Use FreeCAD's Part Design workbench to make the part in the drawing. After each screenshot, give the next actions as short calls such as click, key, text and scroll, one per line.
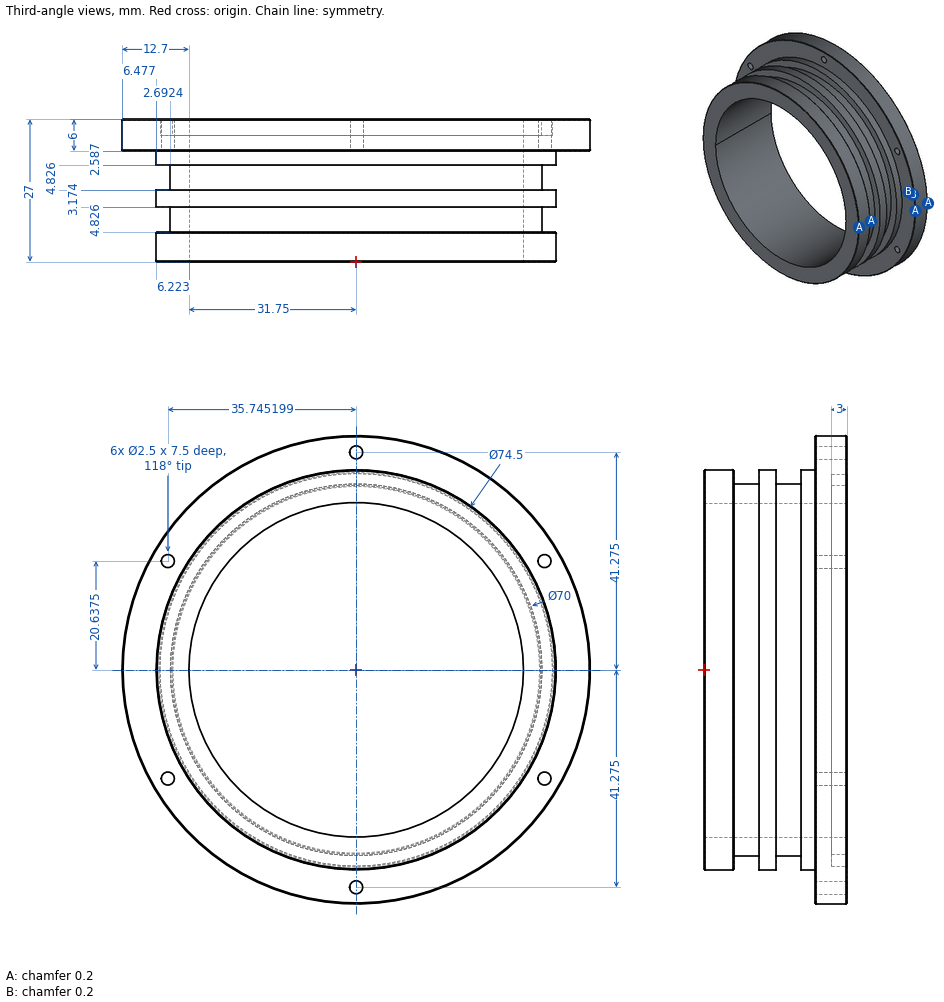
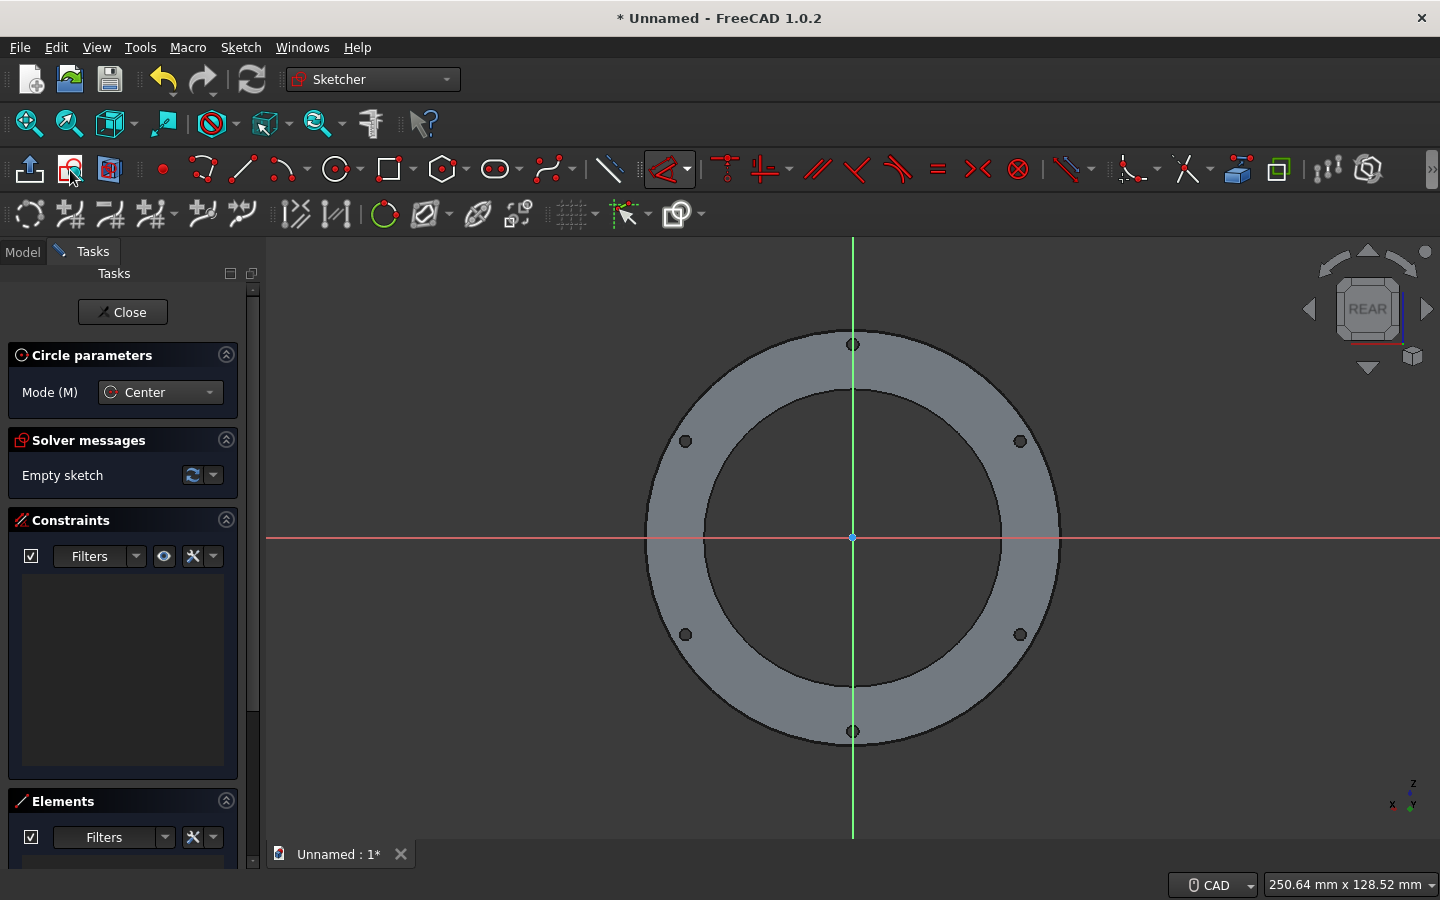
click(853, 538)
move(976, 415)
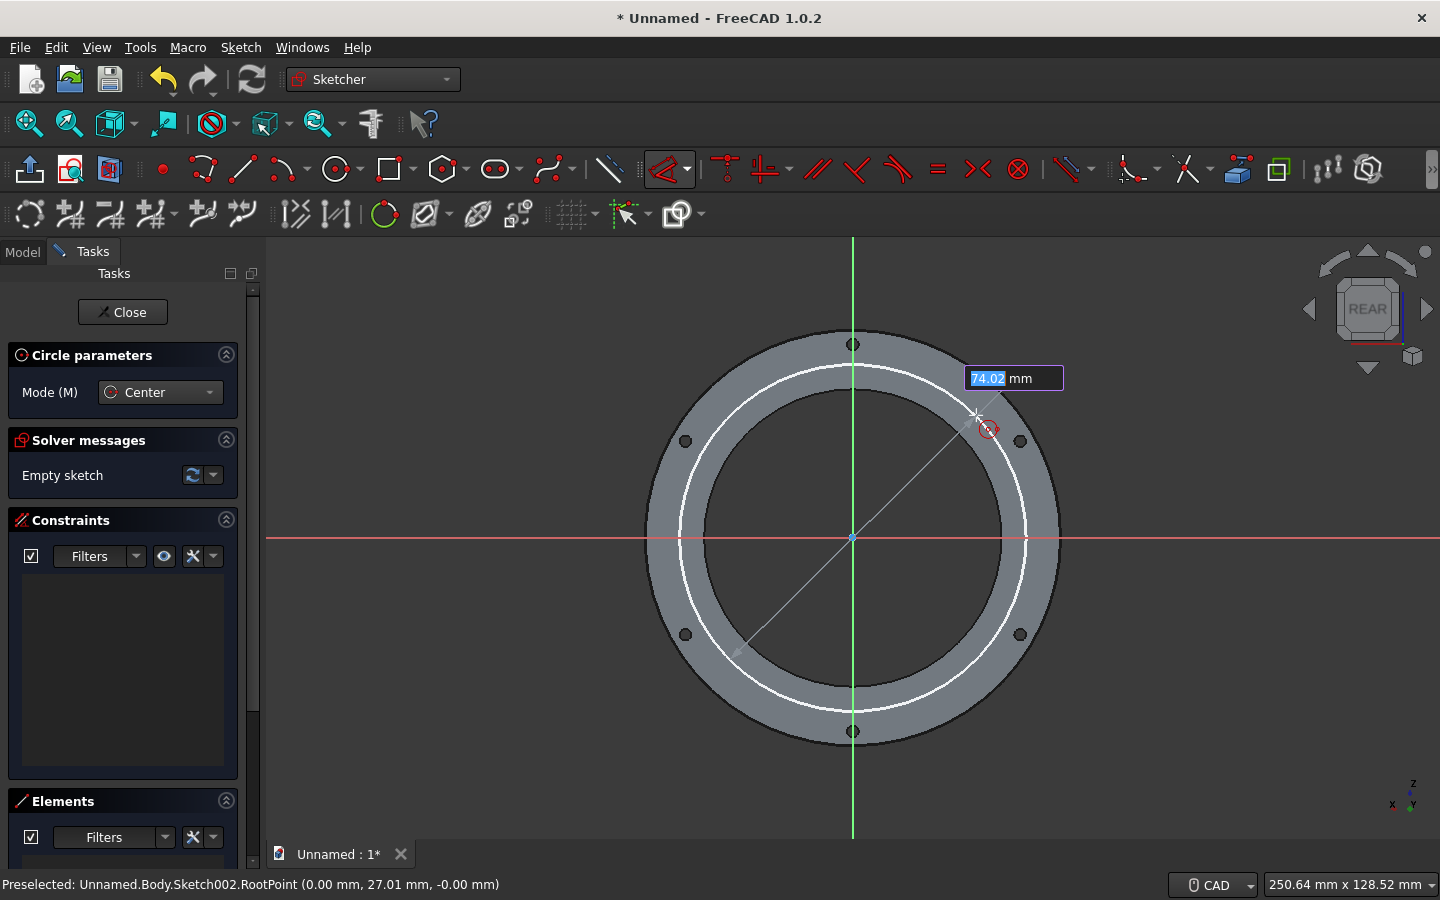
text(74.5)
key(Return)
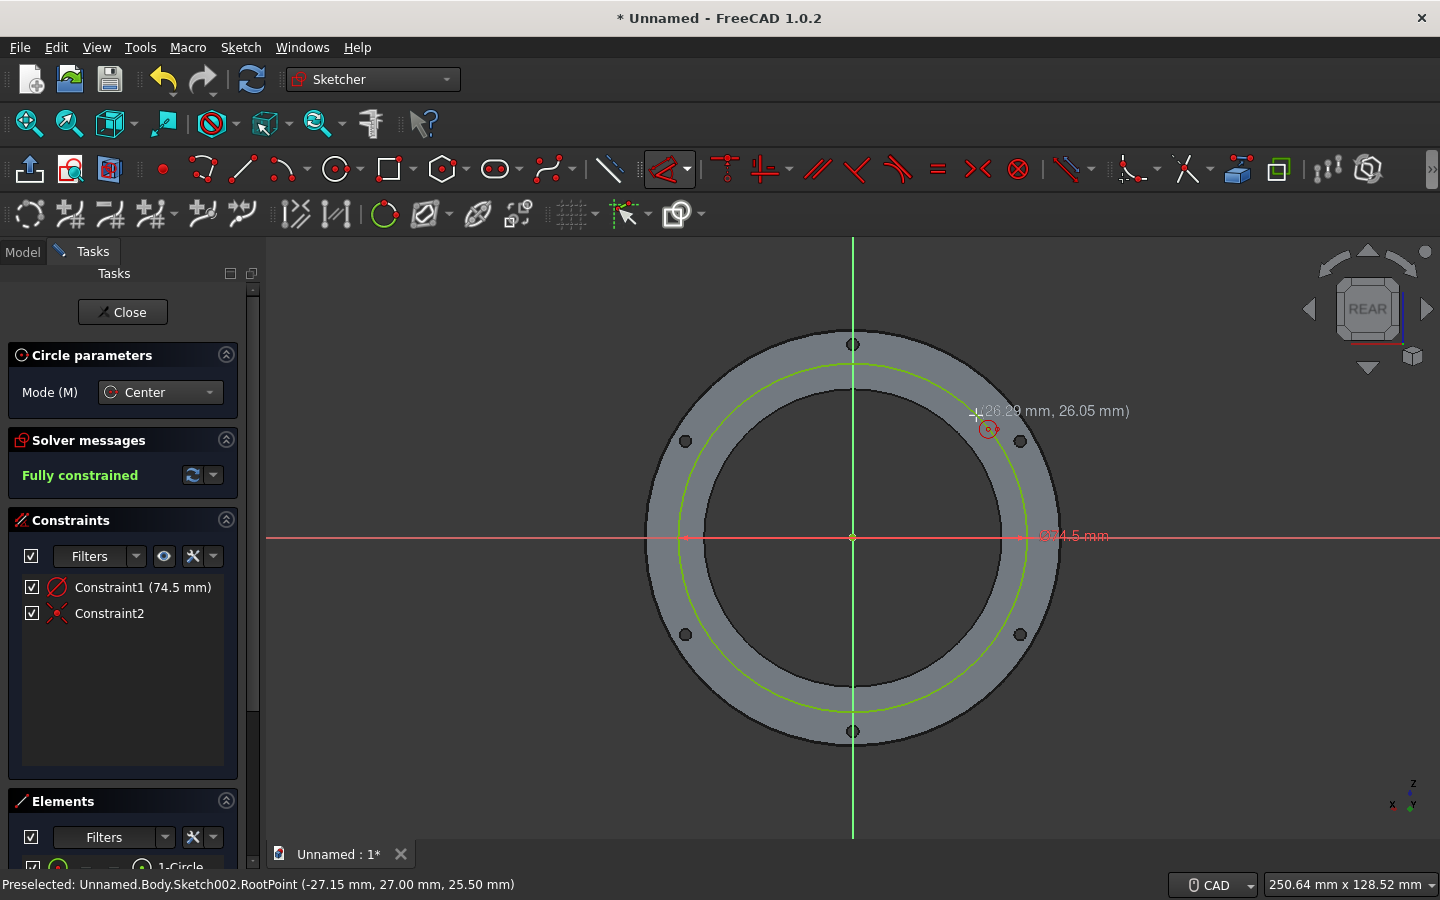
click(853, 538)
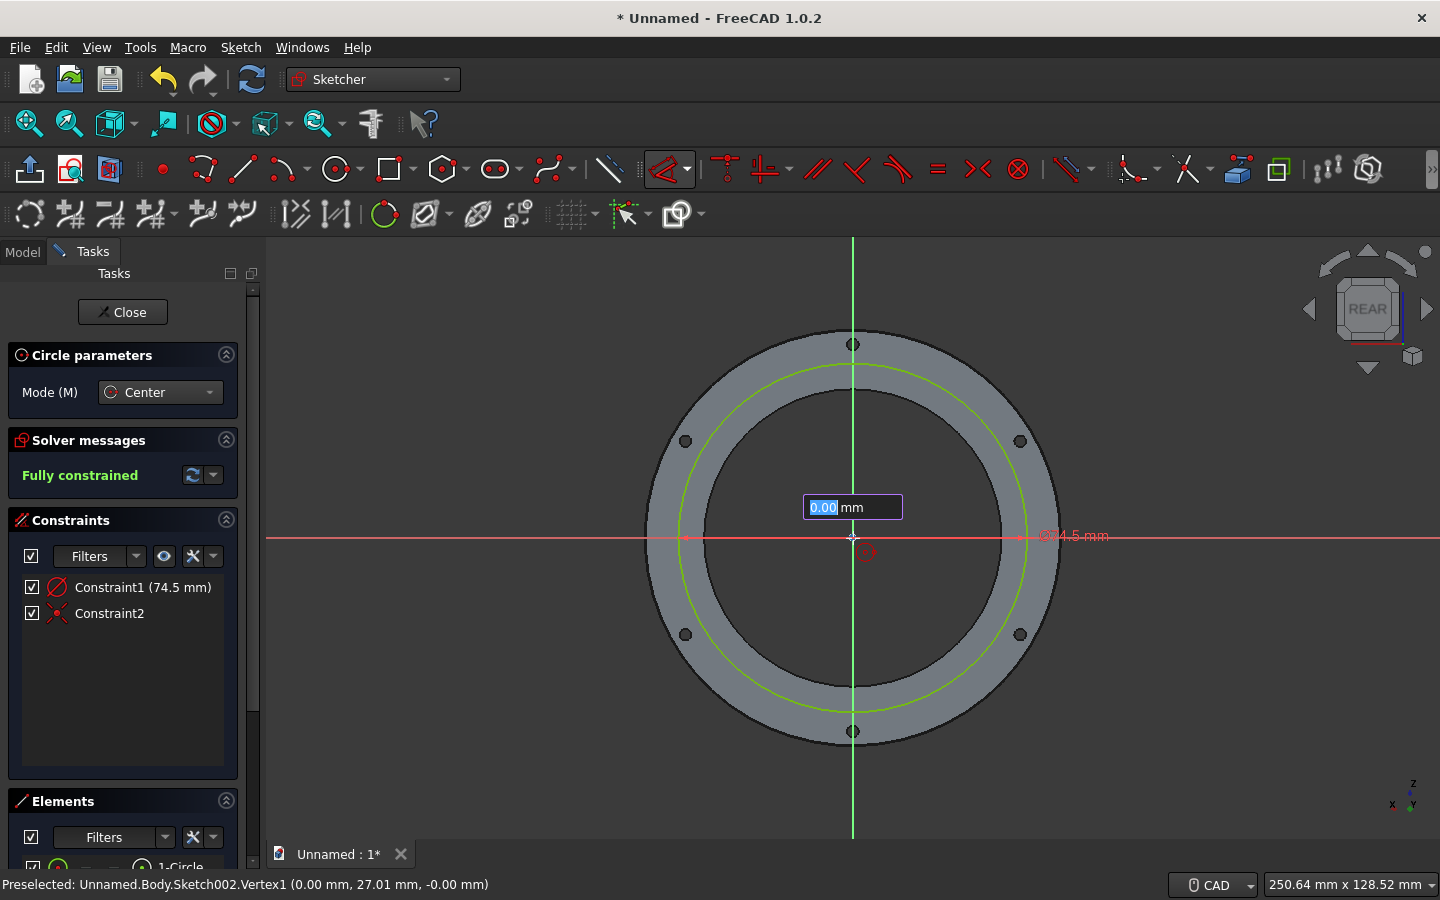
scroll(969, 422, up, 3)
move(968, 422)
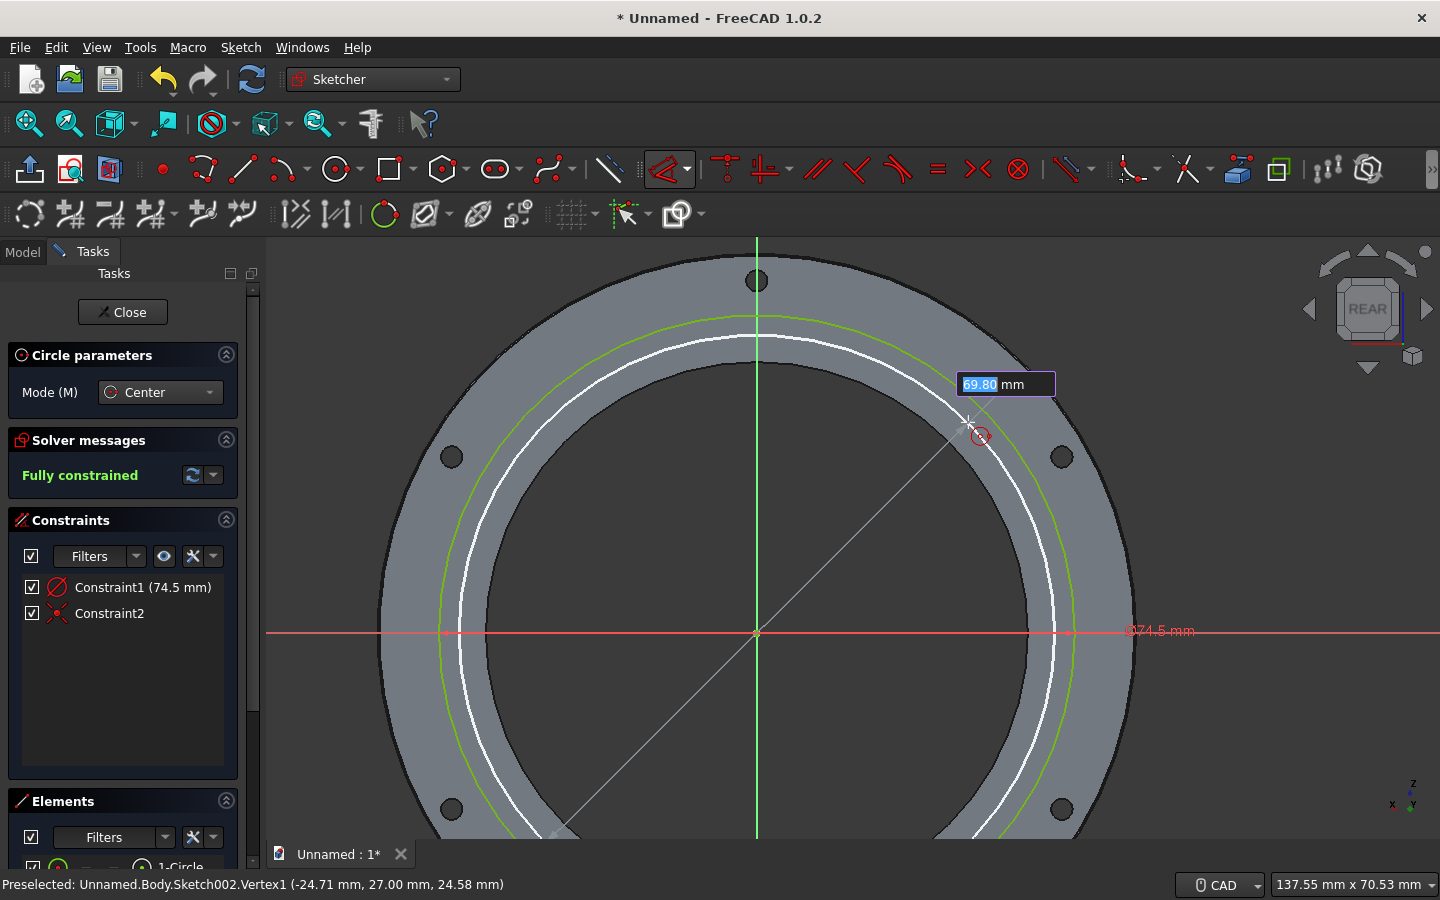
text(70)
key(Return)
key(Escape)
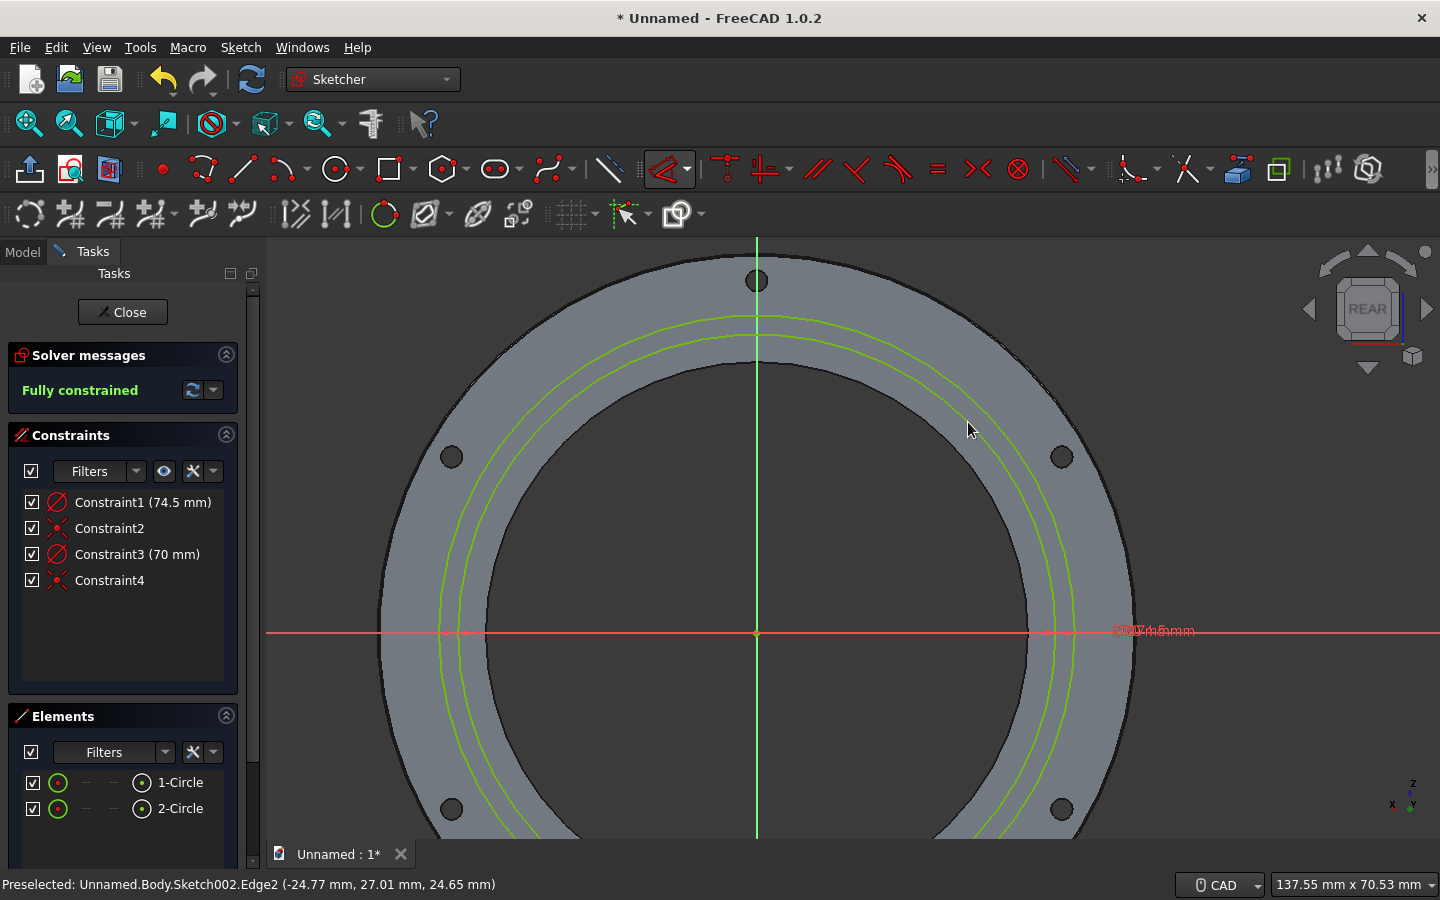
click(123, 312)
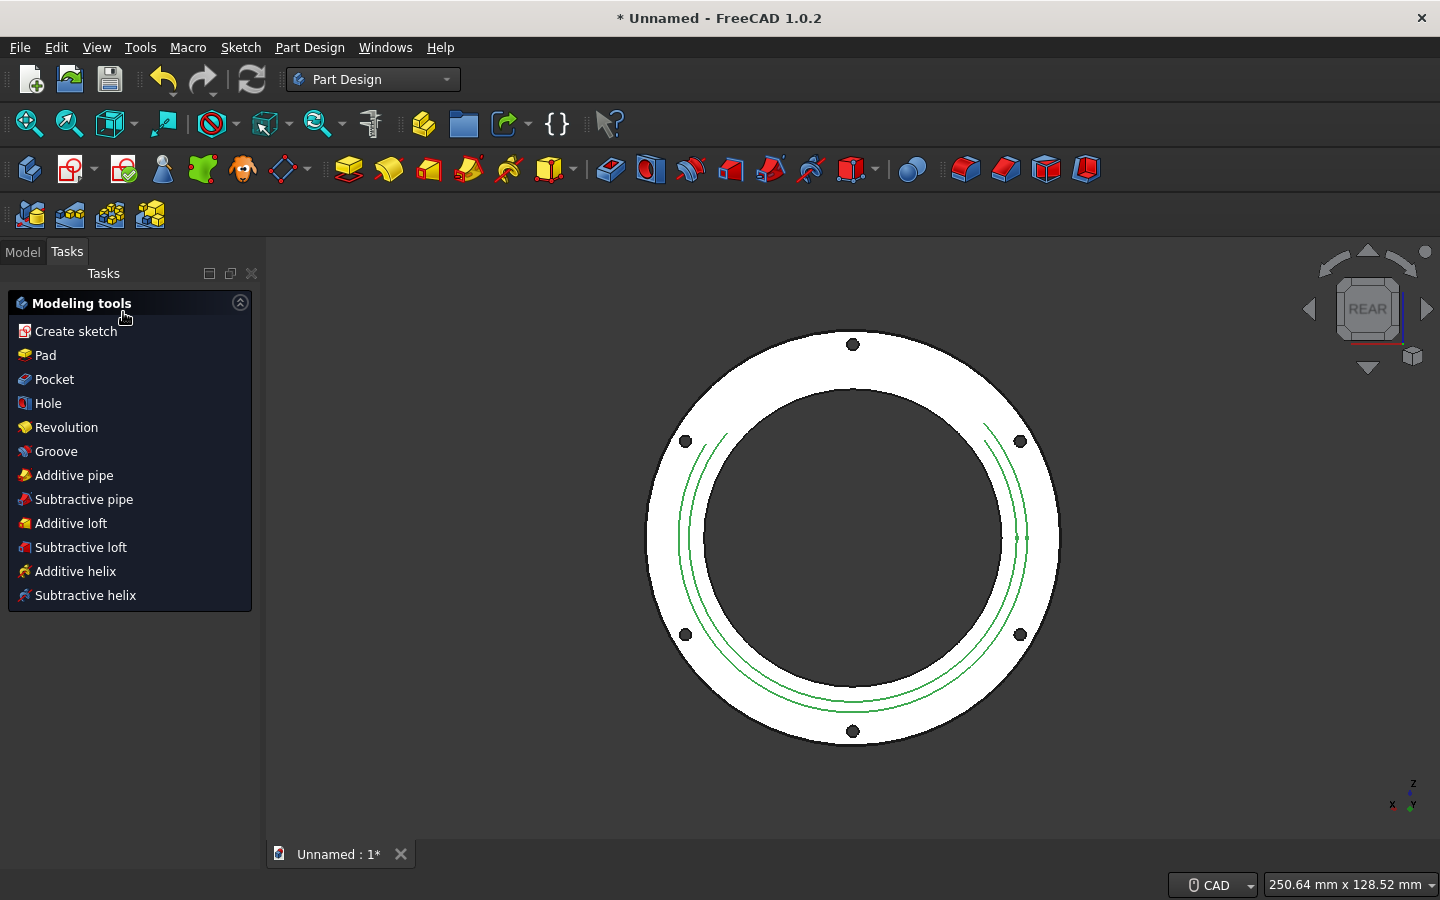
click(612, 170)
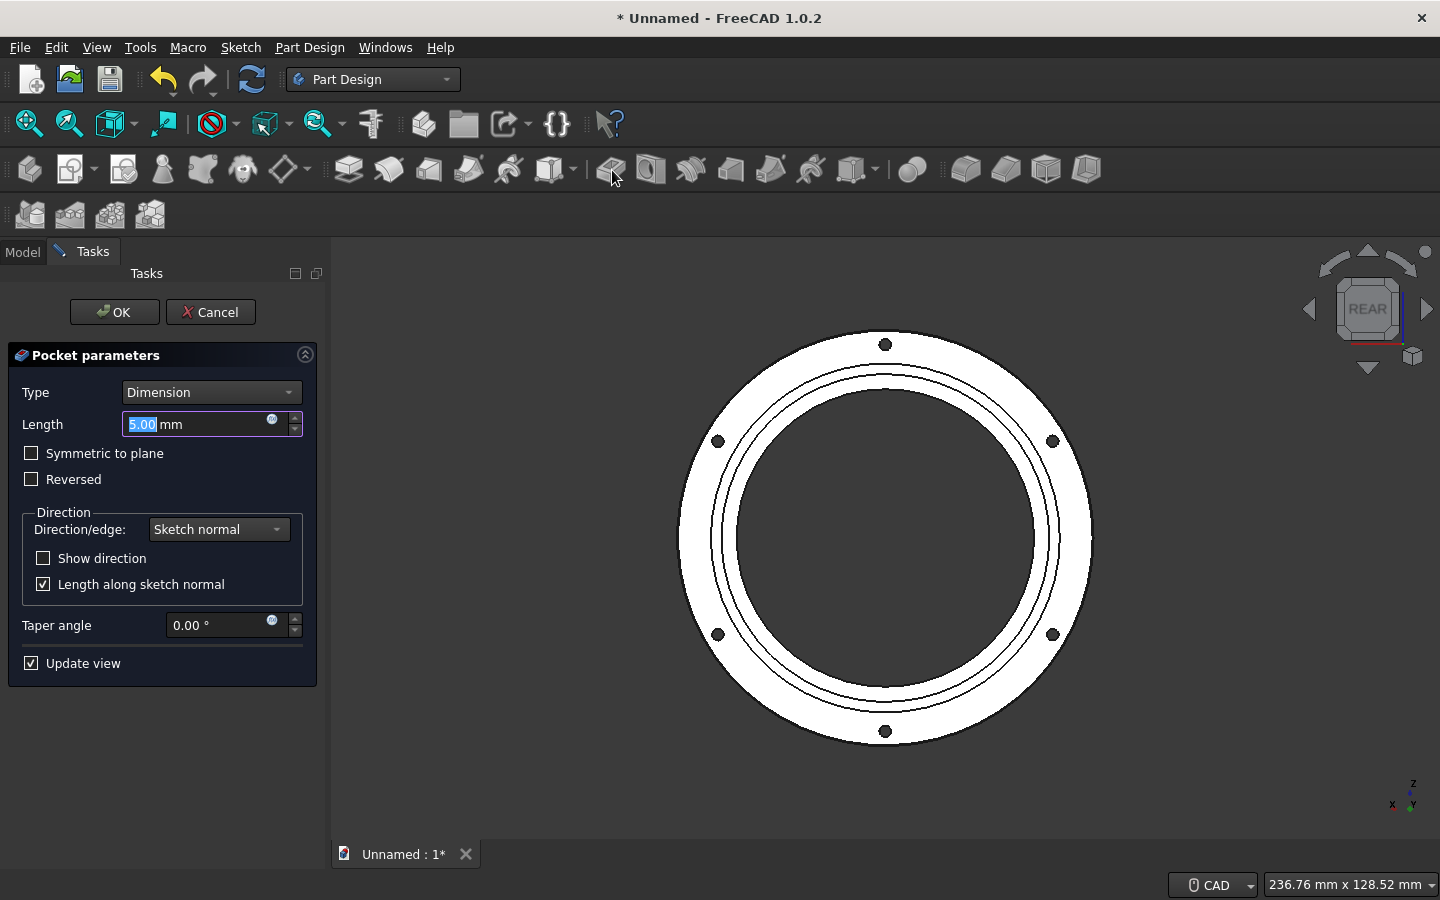
text(3)
key(Tab)